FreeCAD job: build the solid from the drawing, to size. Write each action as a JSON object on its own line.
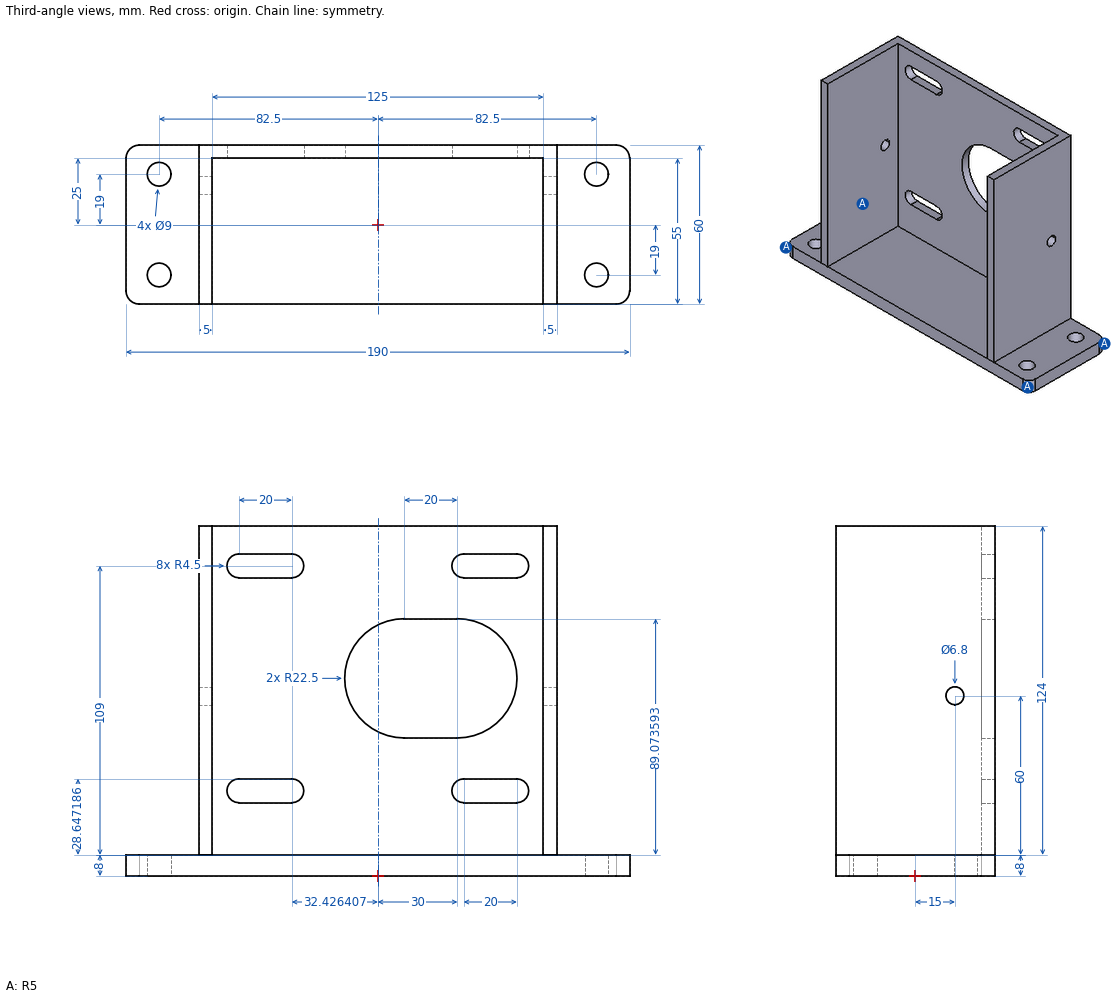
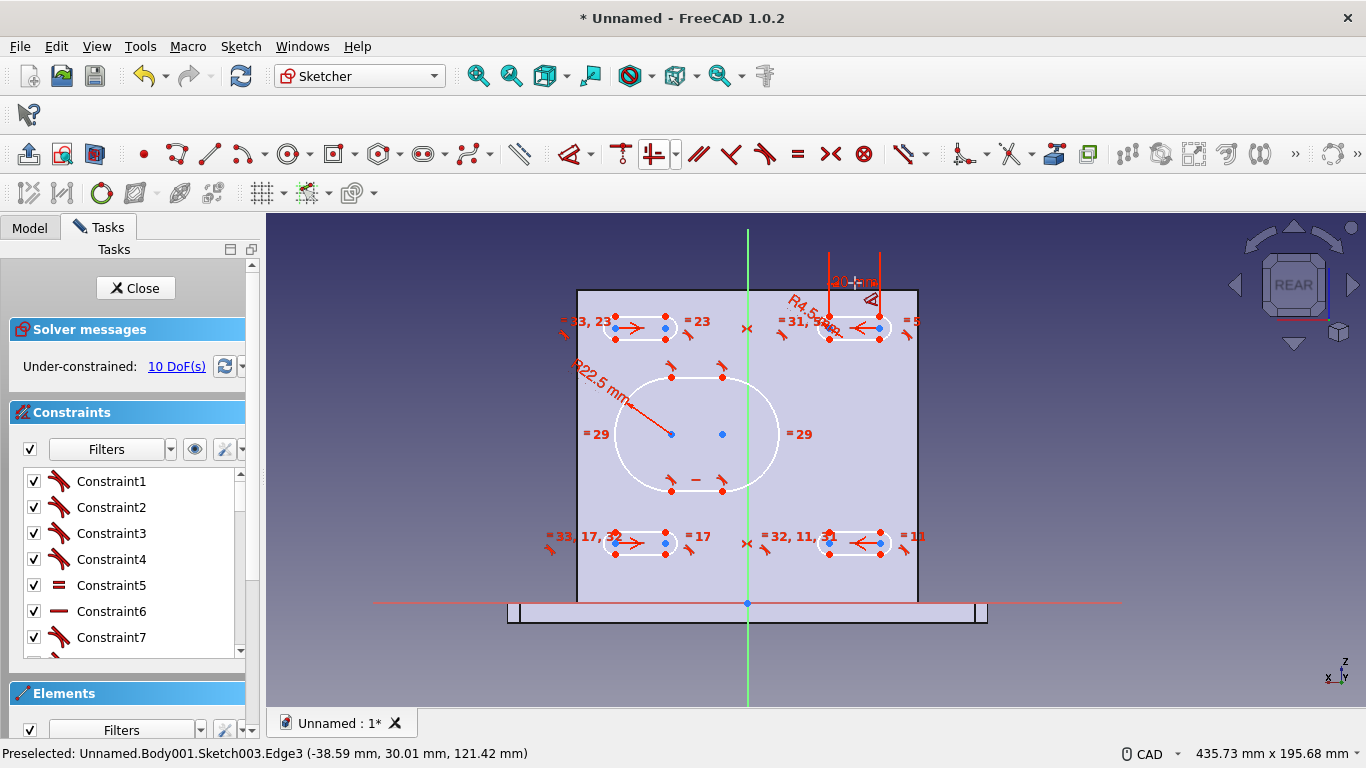
{"action": "left_click", "coordinate": [845, 532]}
{"action": "left_click", "coordinate": [855, 498]}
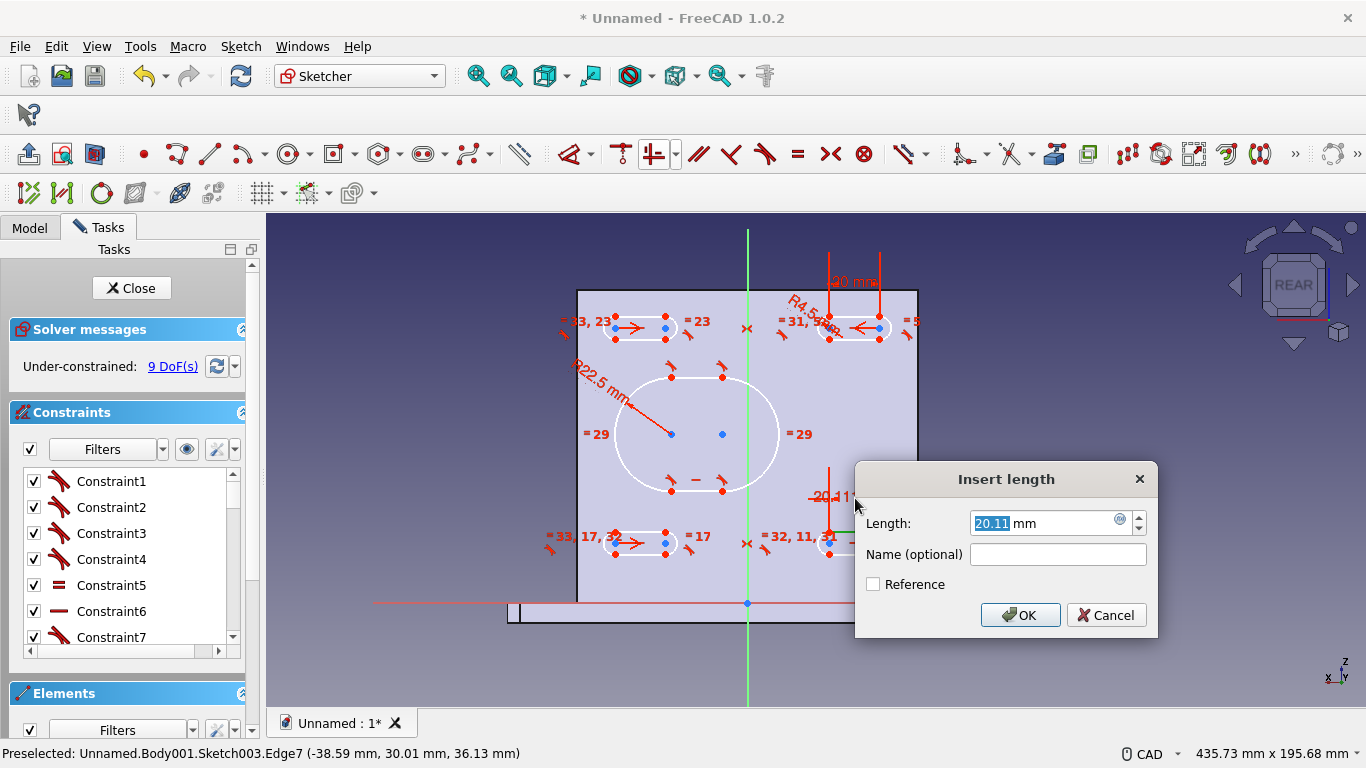
{"action": "type", "text": "20"}
{"action": "key", "text": "Return"}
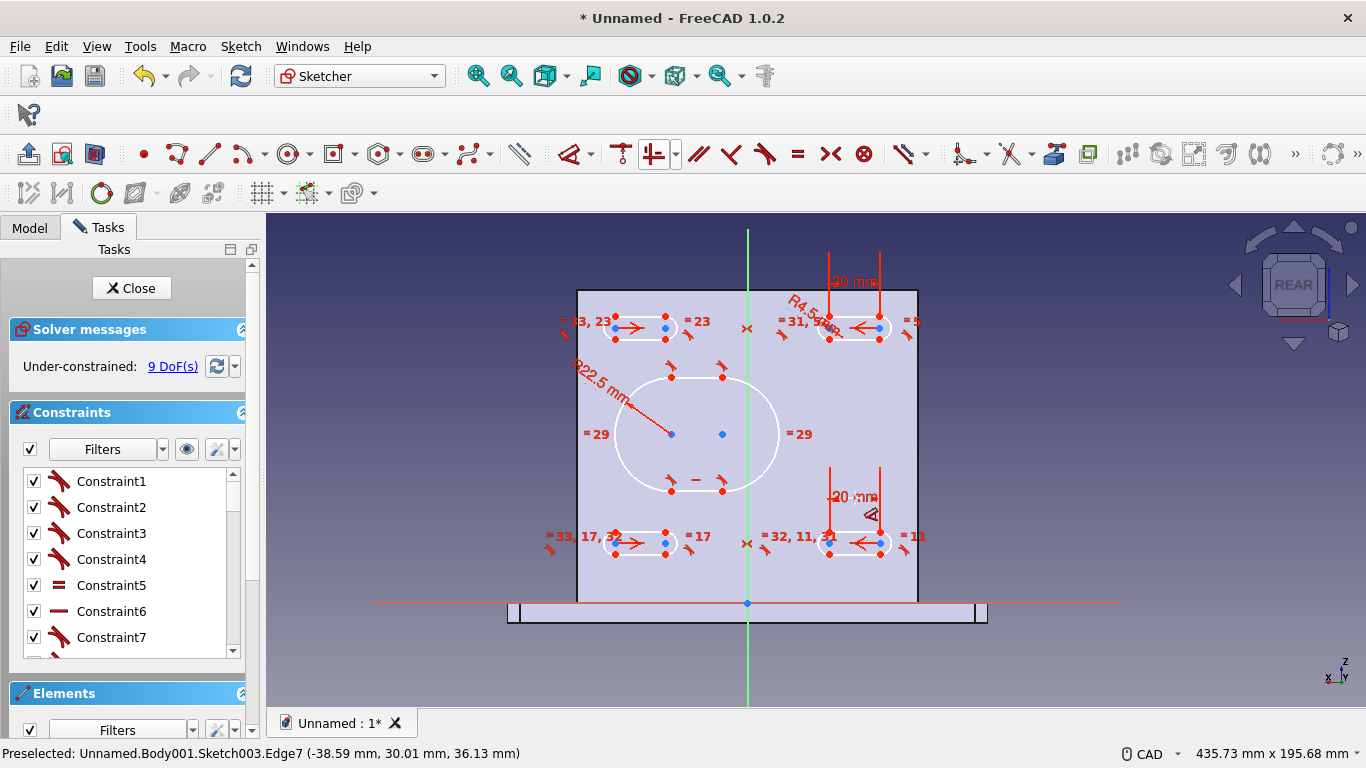
{"action": "left_click", "coordinate": [630, 532]}
{"action": "left_click", "coordinate": [640, 498]}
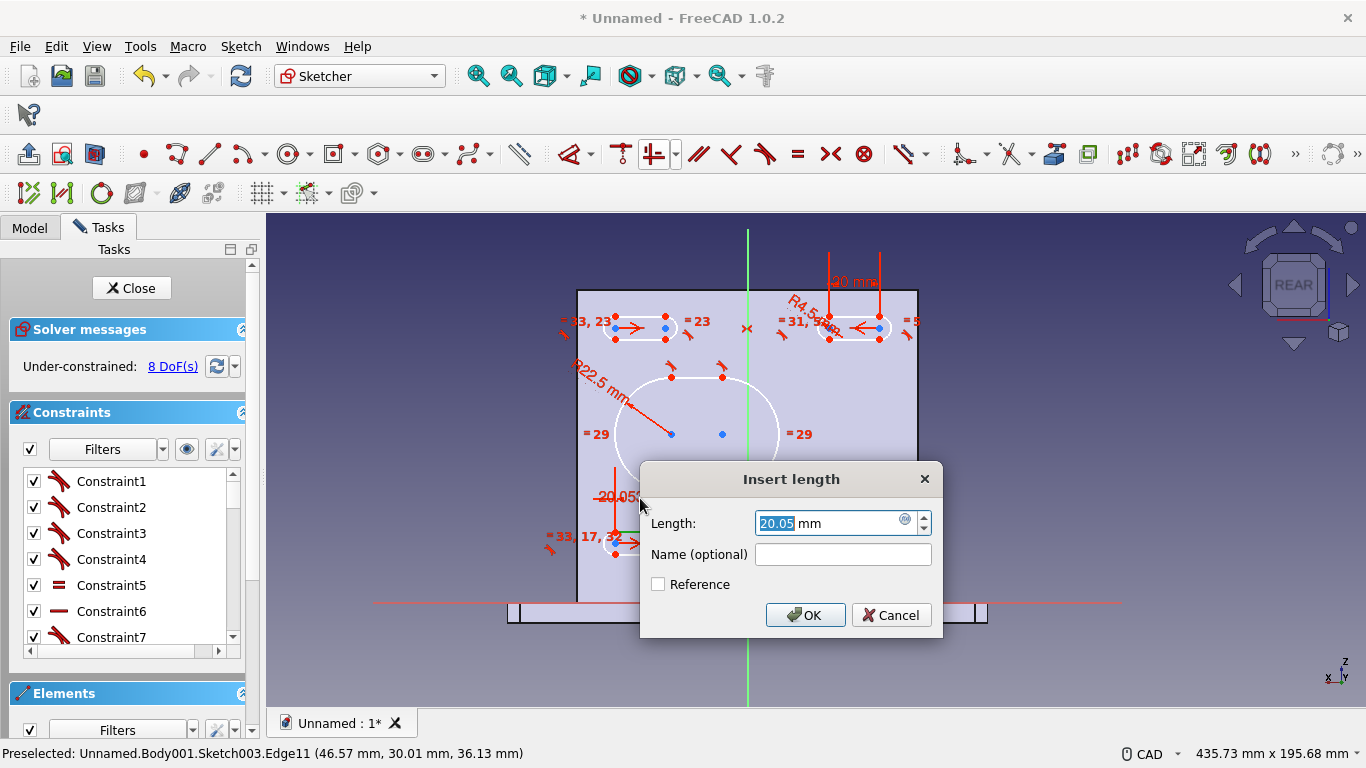
{"action": "type", "text": "20"}
{"action": "key", "text": "Return"}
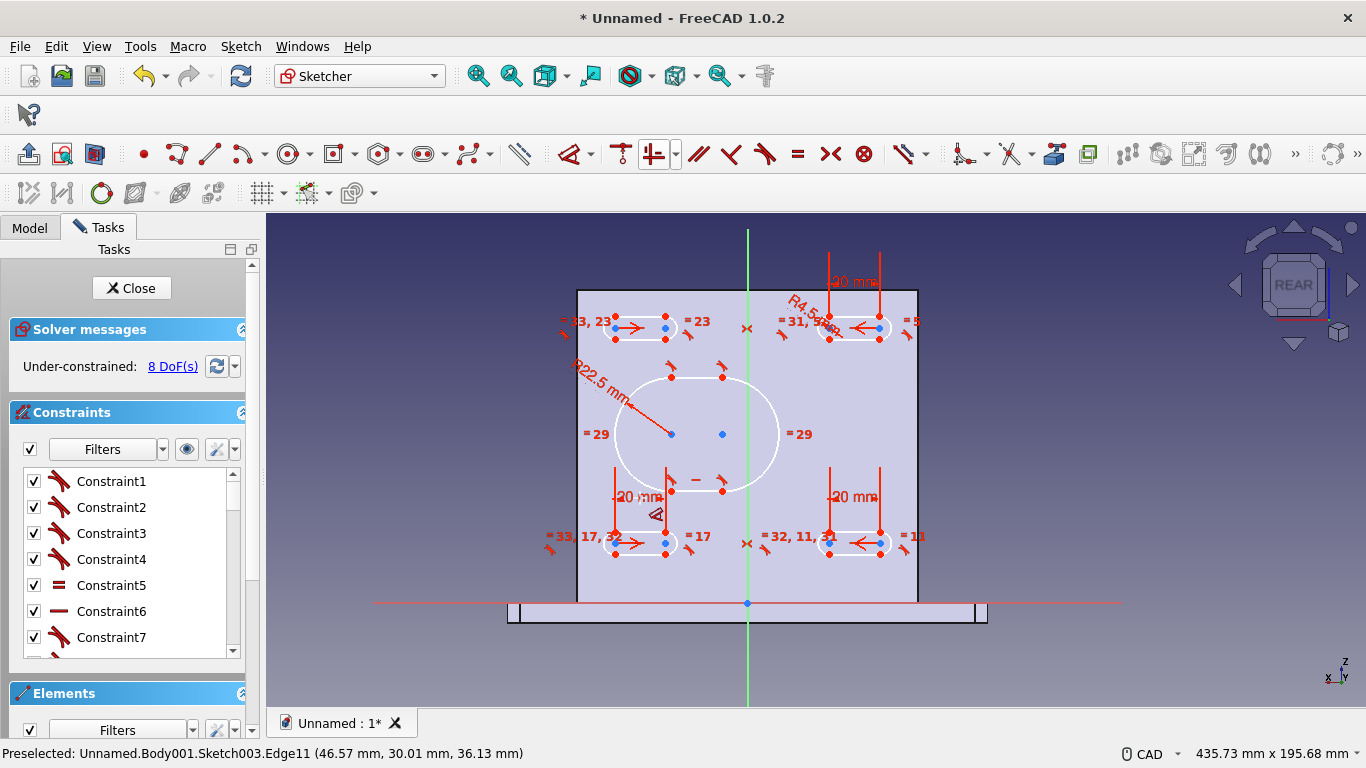
{"action": "left_click", "coordinate": [630, 317]}
{"action": "left_click", "coordinate": [640, 283]}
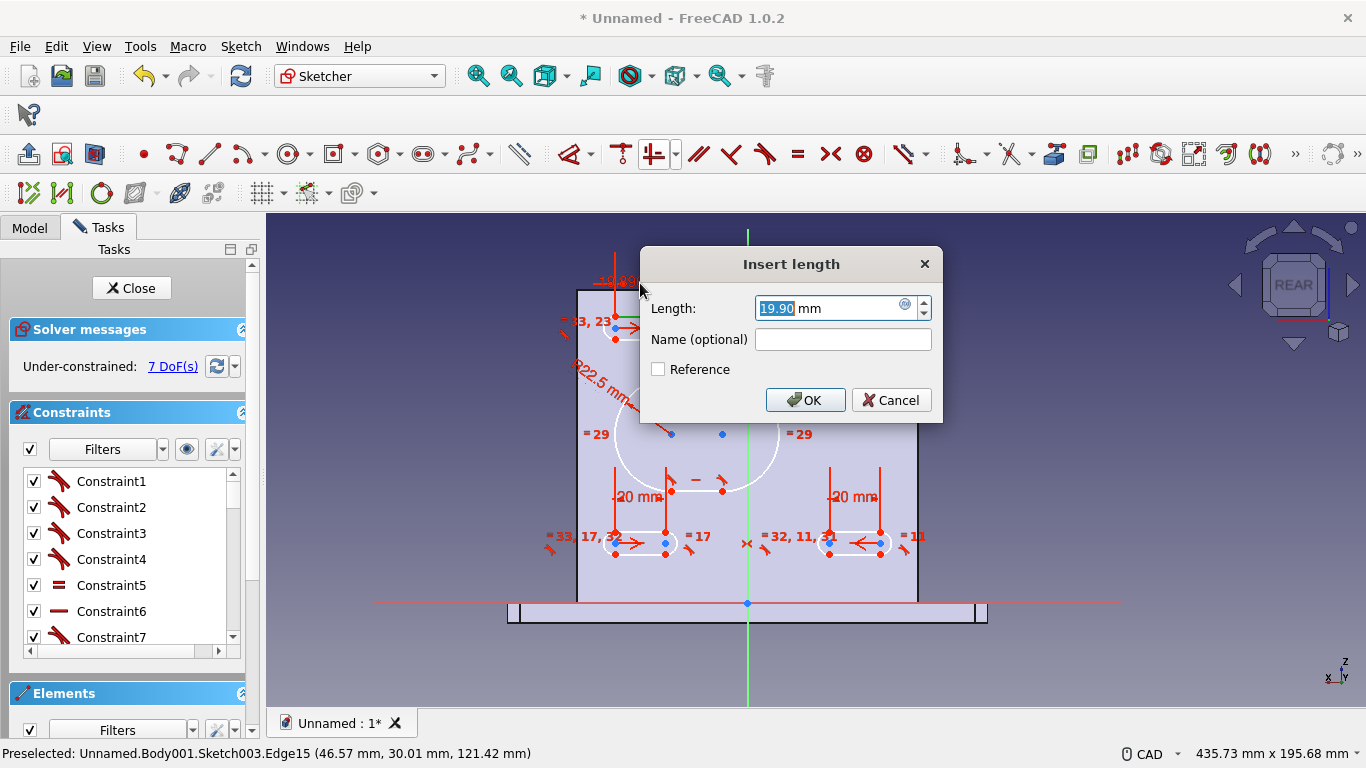
{"action": "type", "text": "20"}
{"action": "key", "text": "Return"}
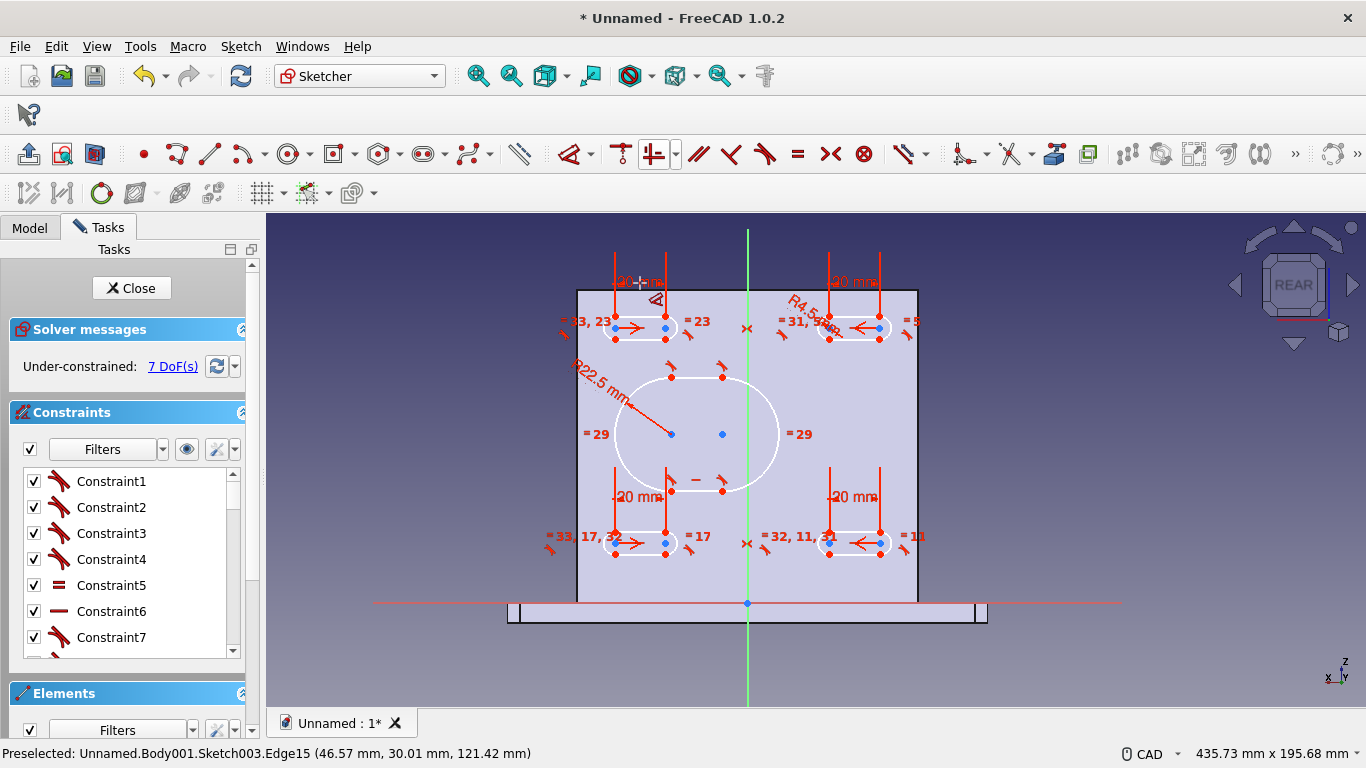
{"action": "left_click", "coordinate": [687, 378]}
{"action": "left_click", "coordinate": [697, 344]}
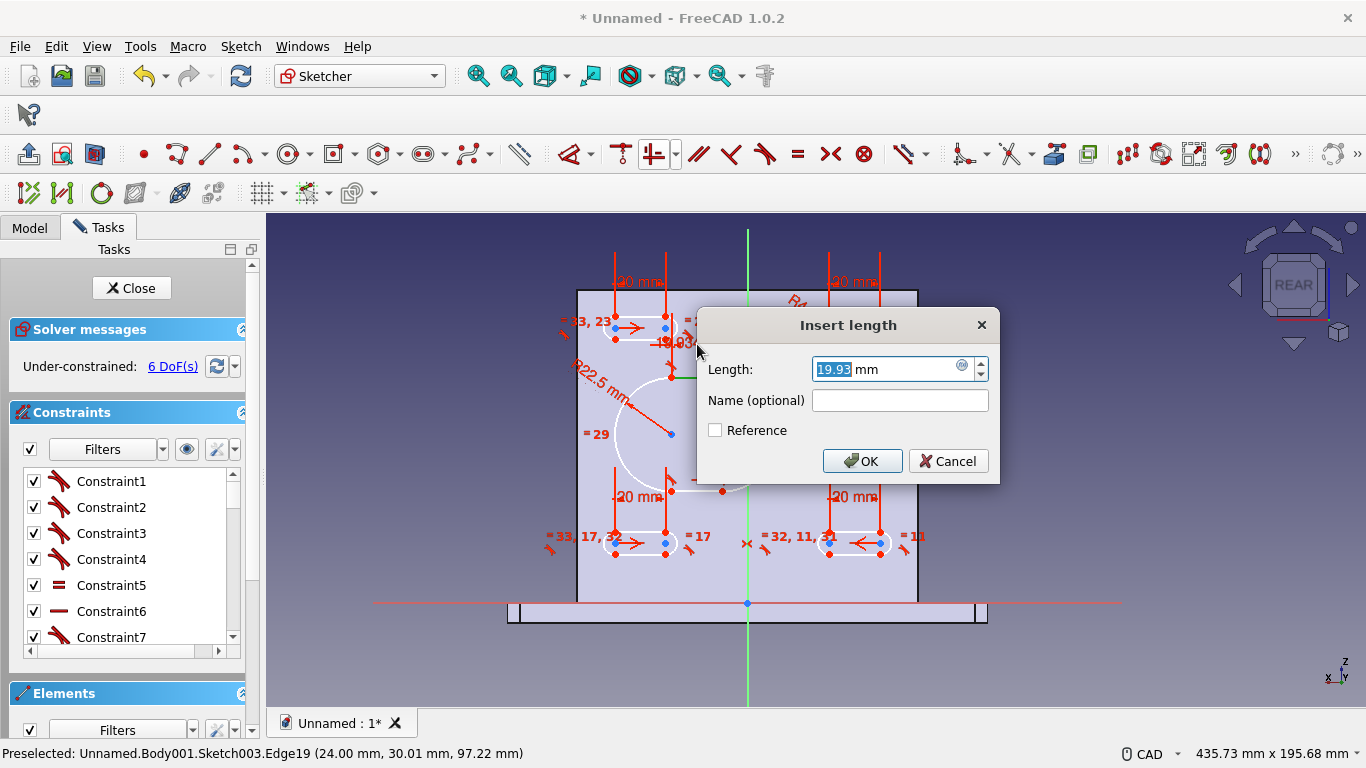
{"action": "type", "text": "20"}
{"action": "key", "text": "Return"}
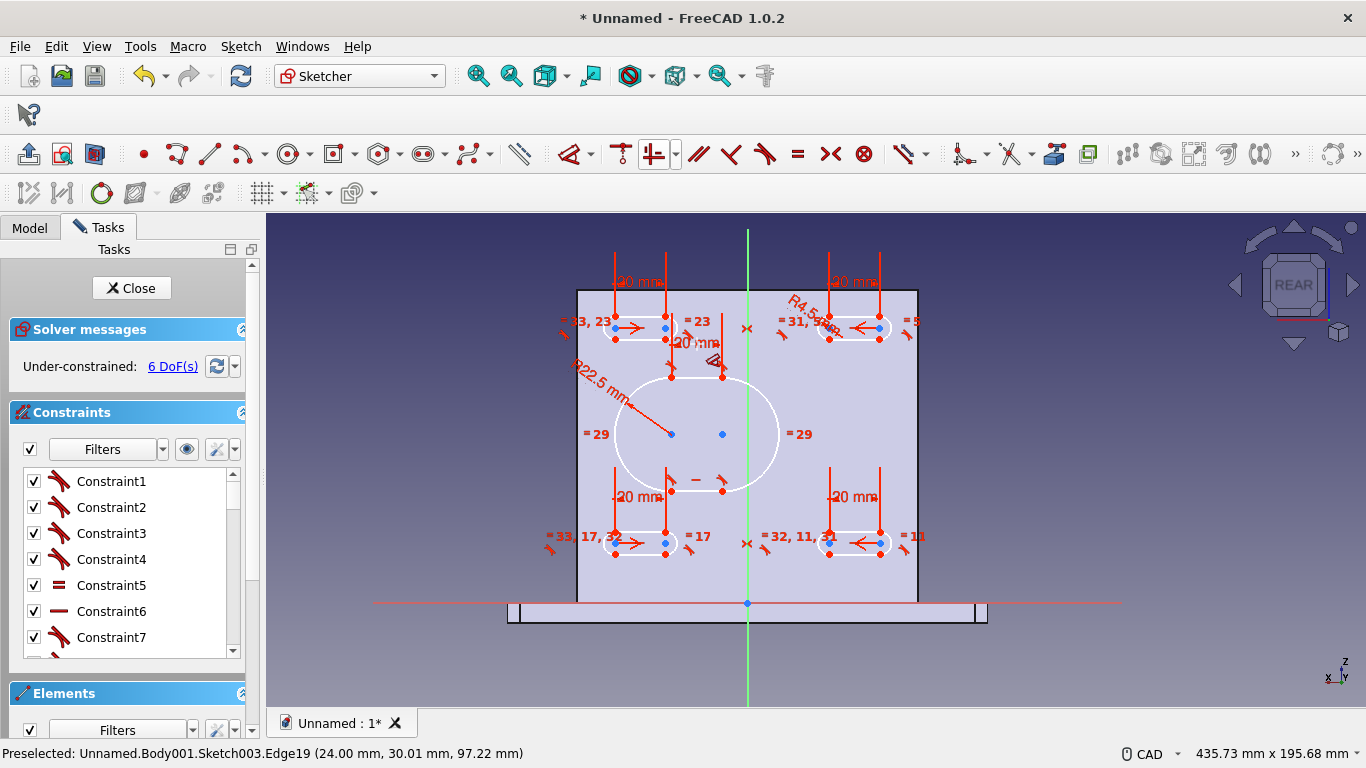
{"action": "left_click", "coordinate": [672, 378]}
{"action": "left_click", "coordinate": [710, 637]}